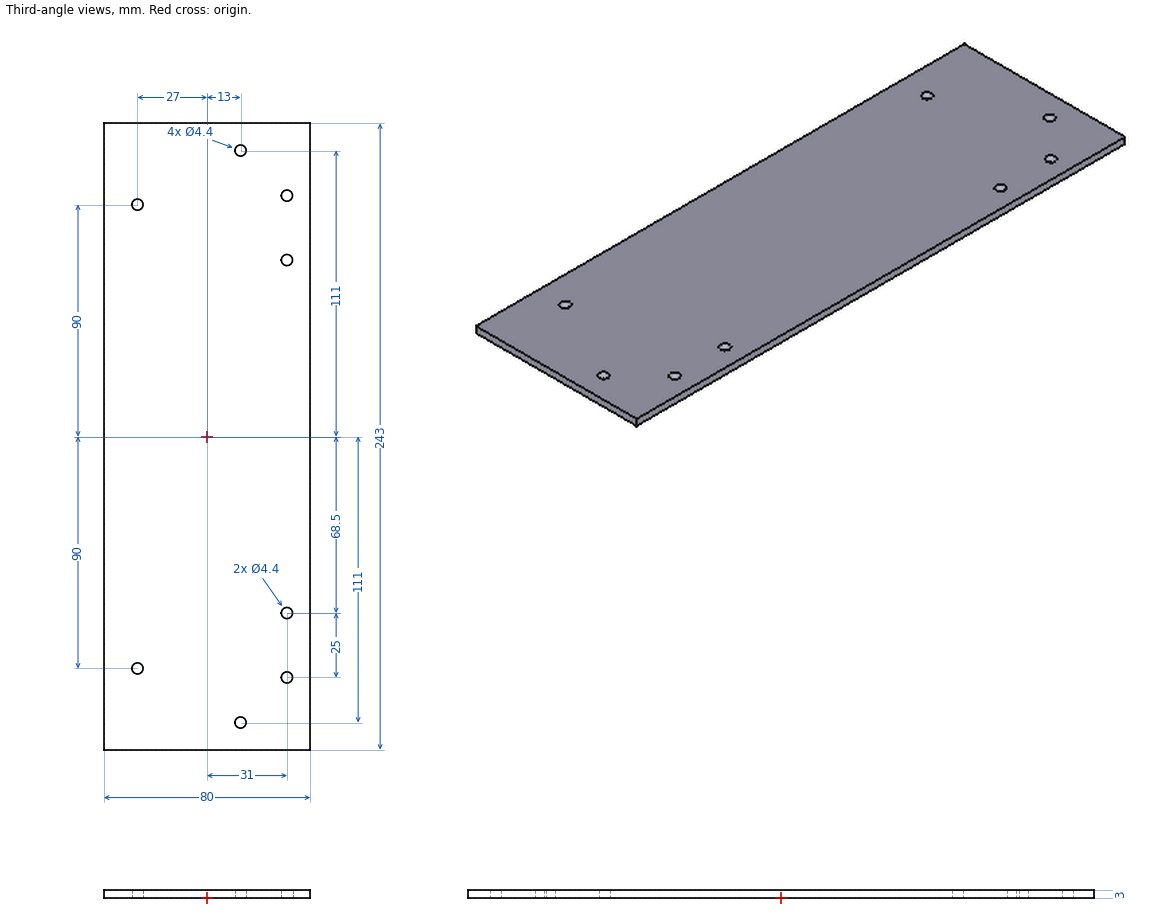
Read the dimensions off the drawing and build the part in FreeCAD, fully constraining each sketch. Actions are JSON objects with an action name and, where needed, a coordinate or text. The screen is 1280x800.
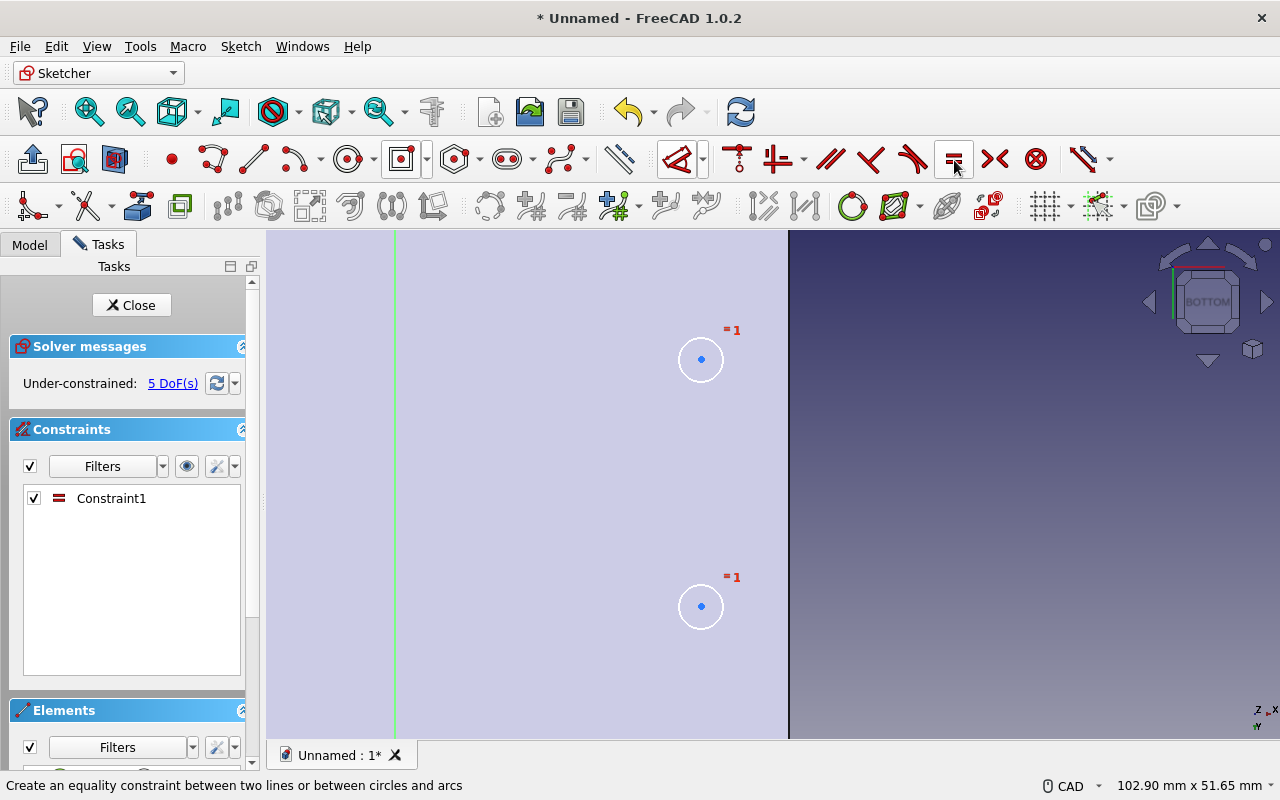
{"action": "left_click", "coordinate": [701, 607]}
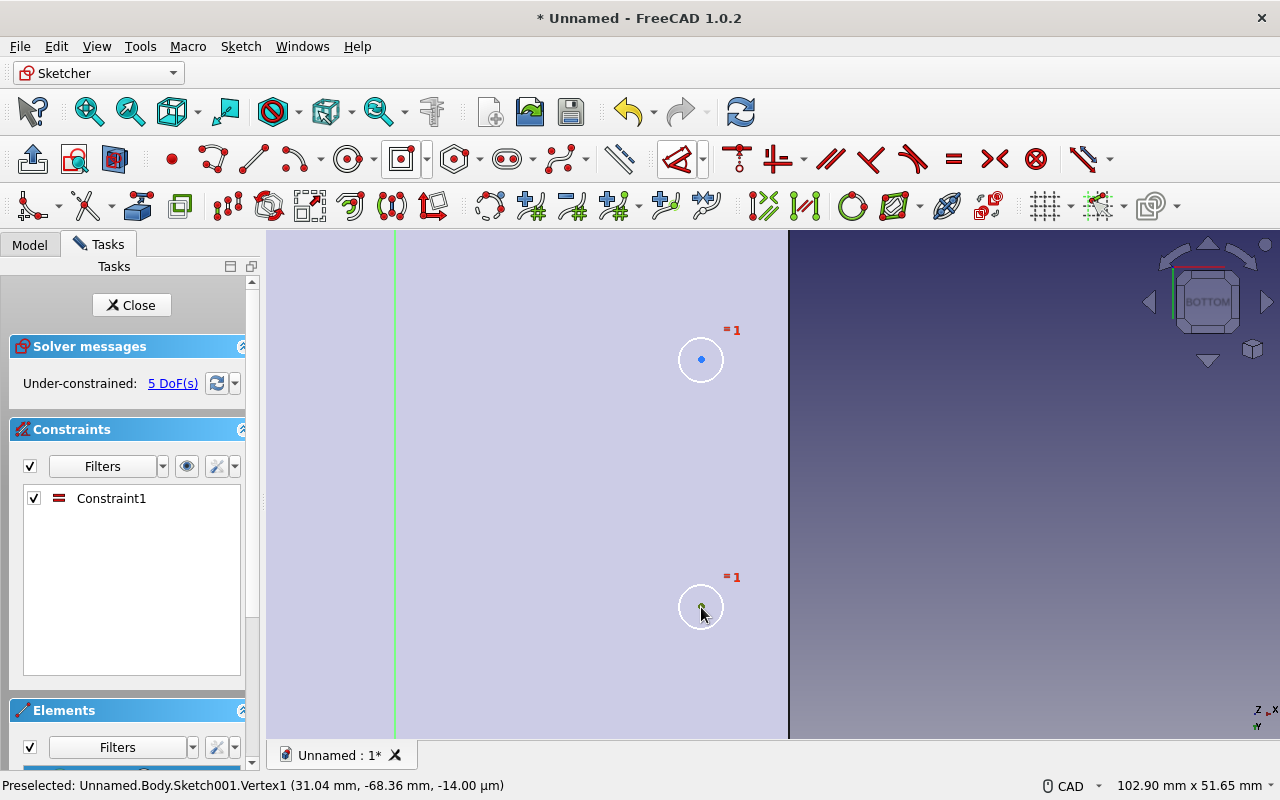
{"action": "left_click", "coordinate": [701, 360]}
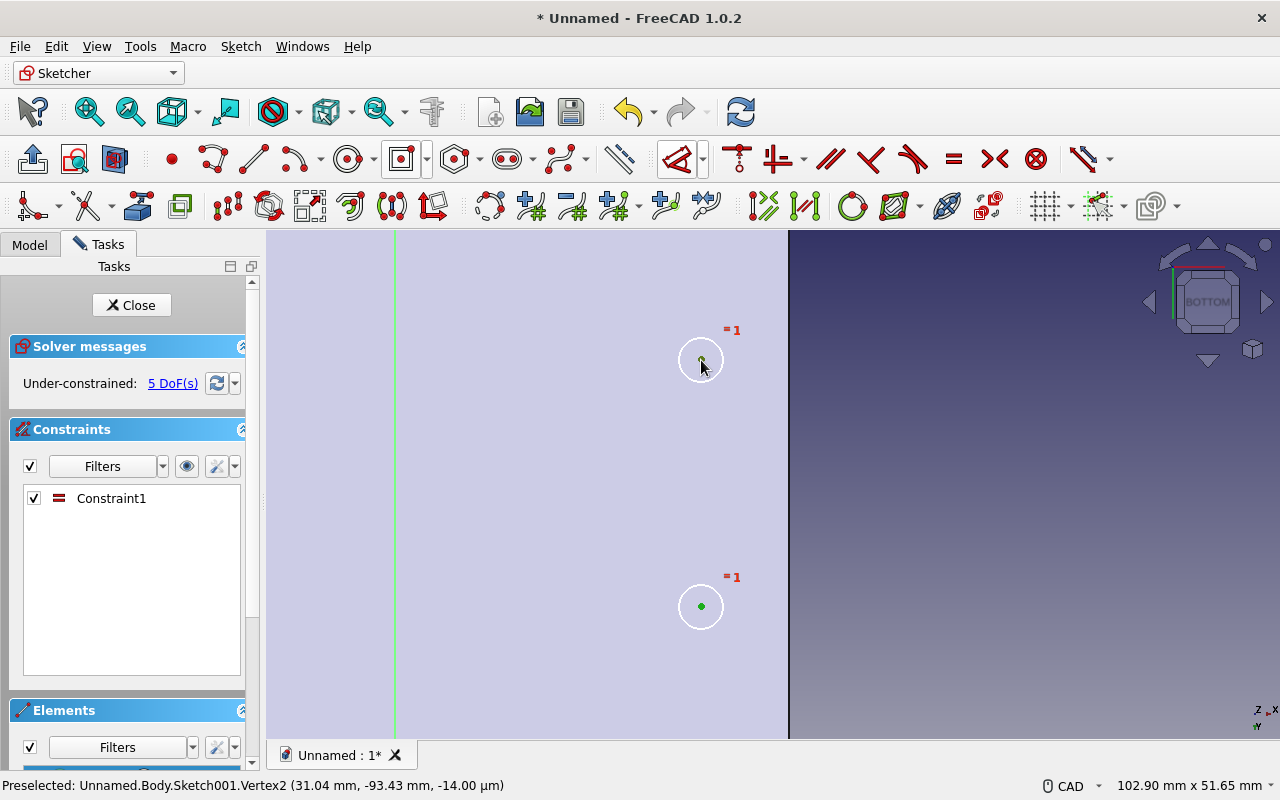
{"action": "left_click", "coordinate": [804, 160]}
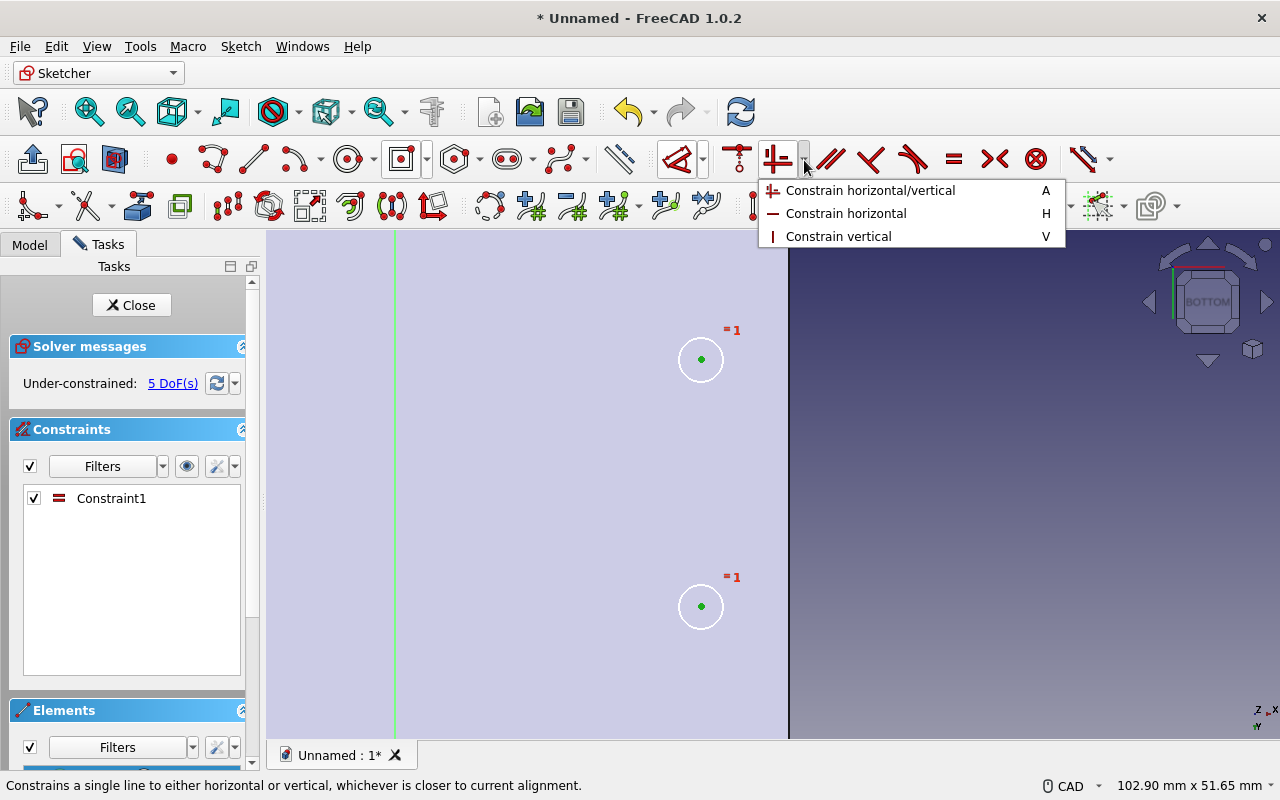
{"action": "left_click", "coordinate": [912, 236]}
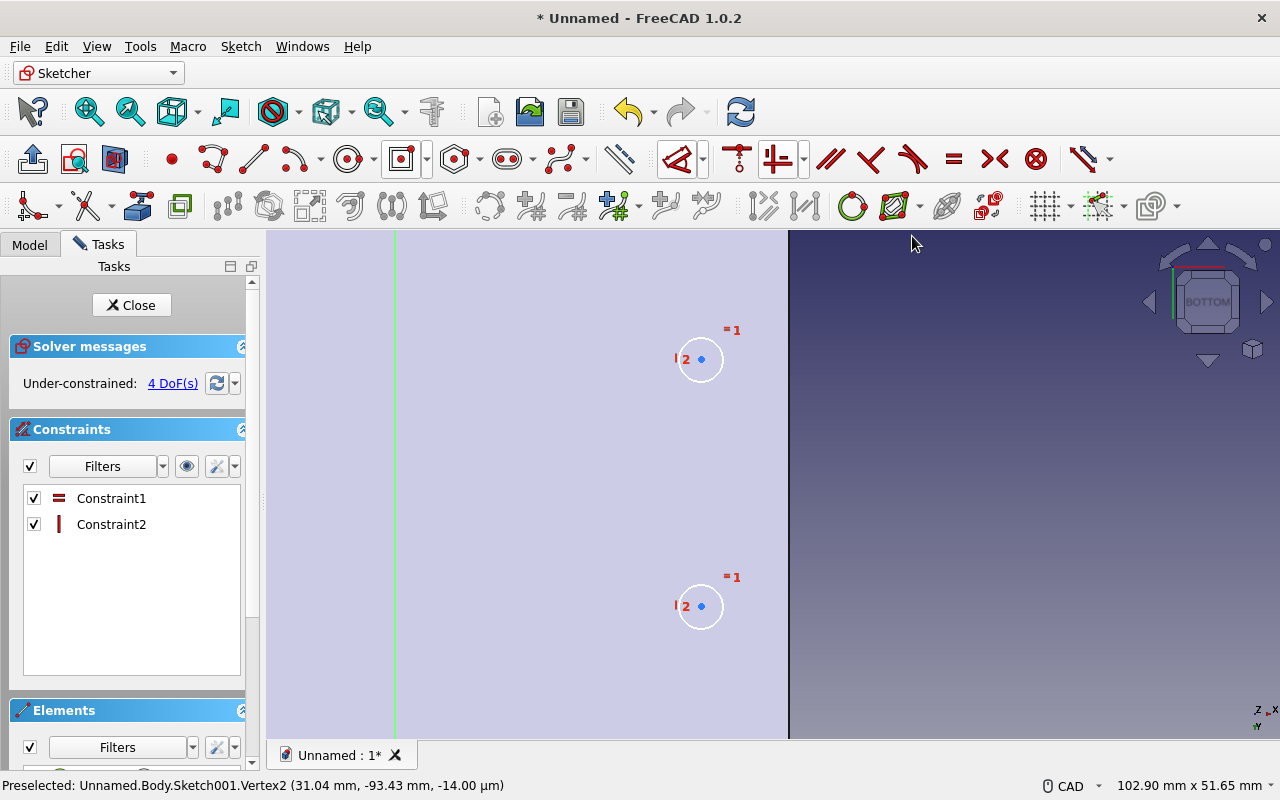
{"action": "left_click", "coordinate": [716, 591]}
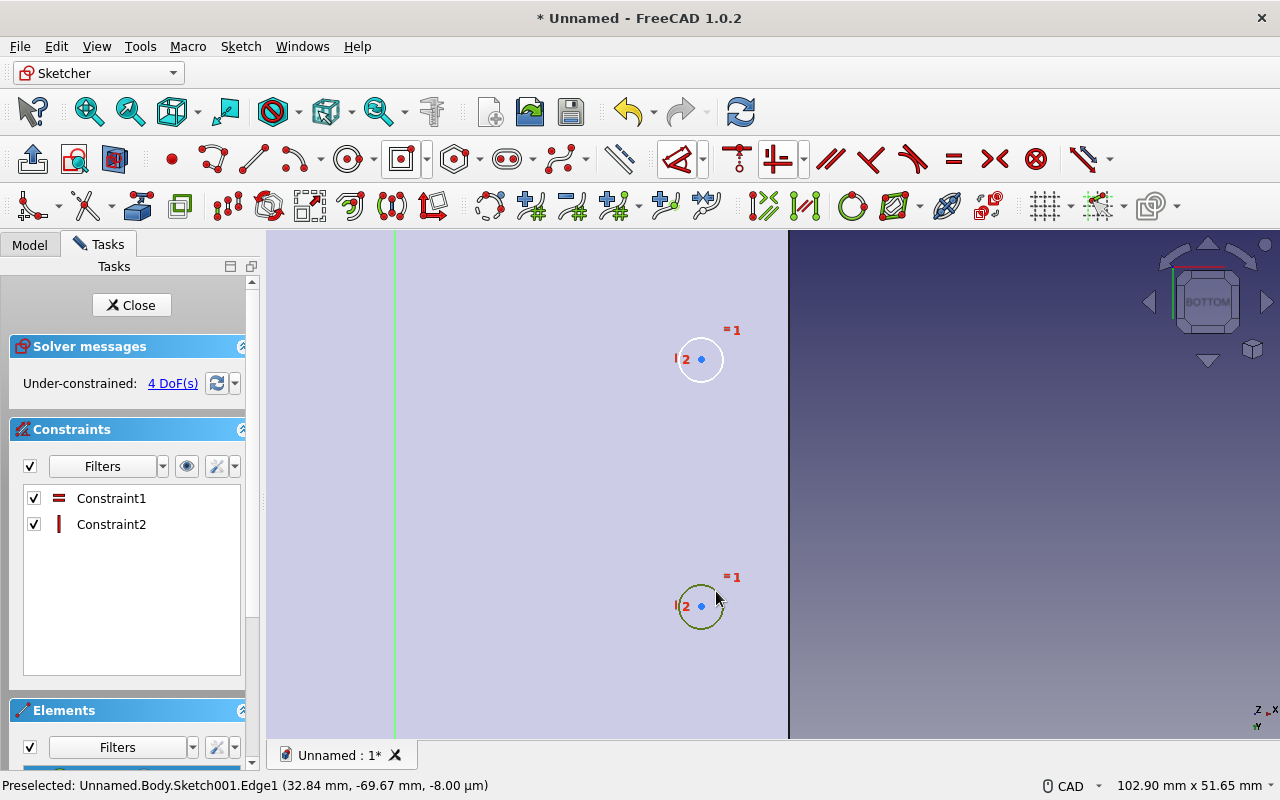
{"action": "left_click", "coordinate": [702, 160]}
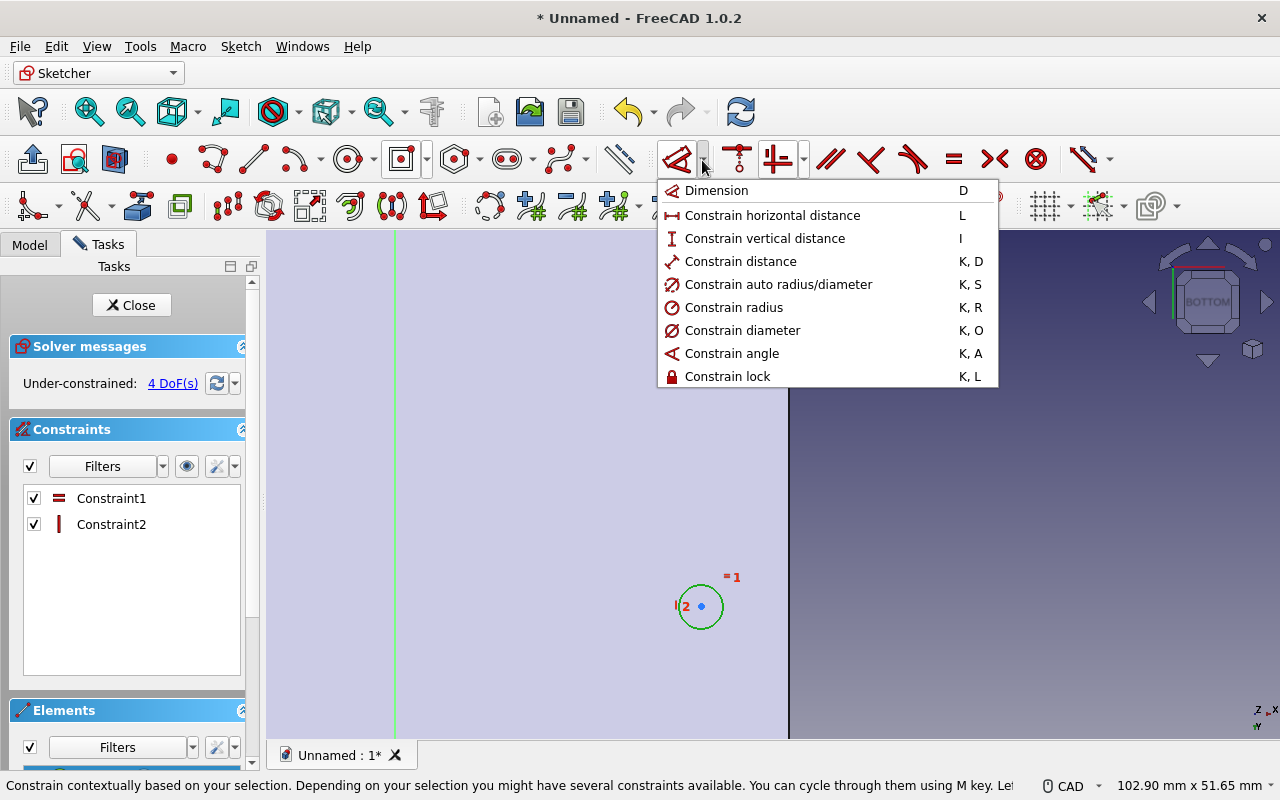
{"action": "left_click", "coordinate": [828, 330]}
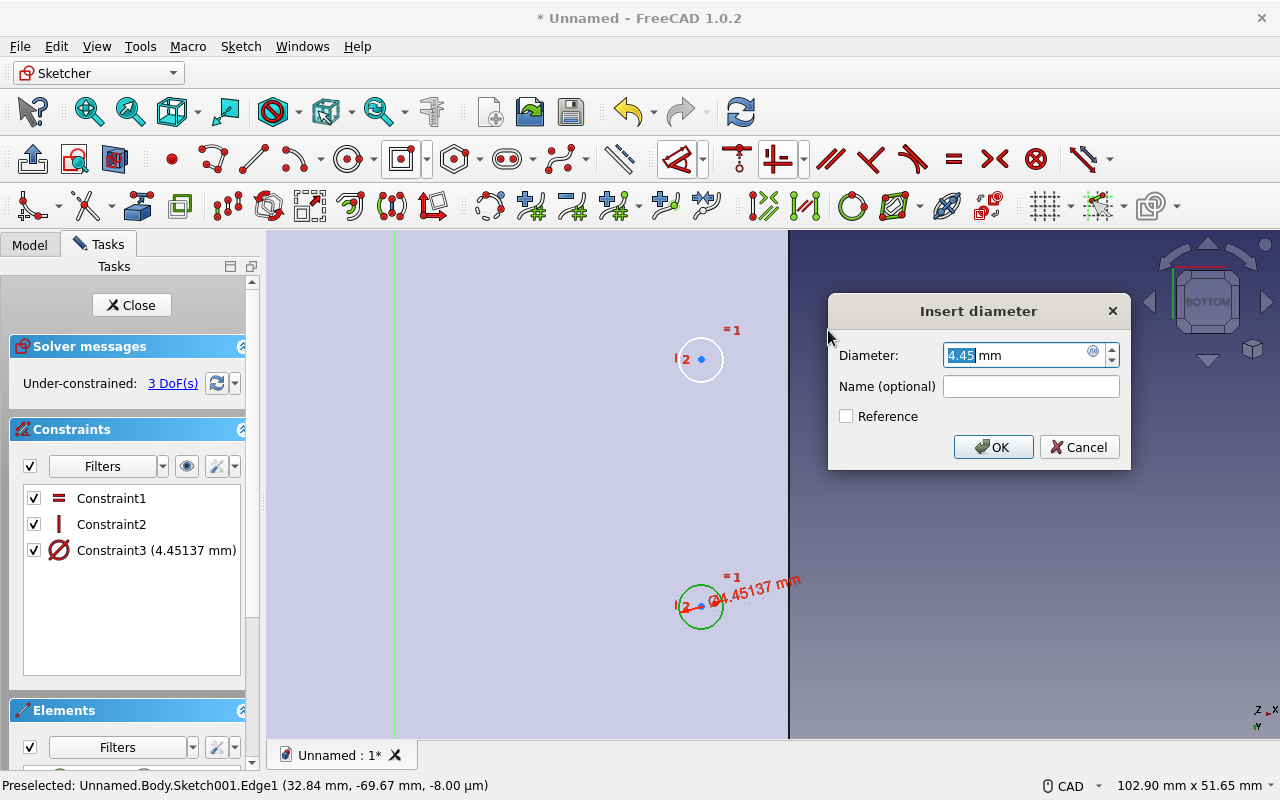
{"action": "type", "text": "4.4"}
{"action": "key", "text": "Return"}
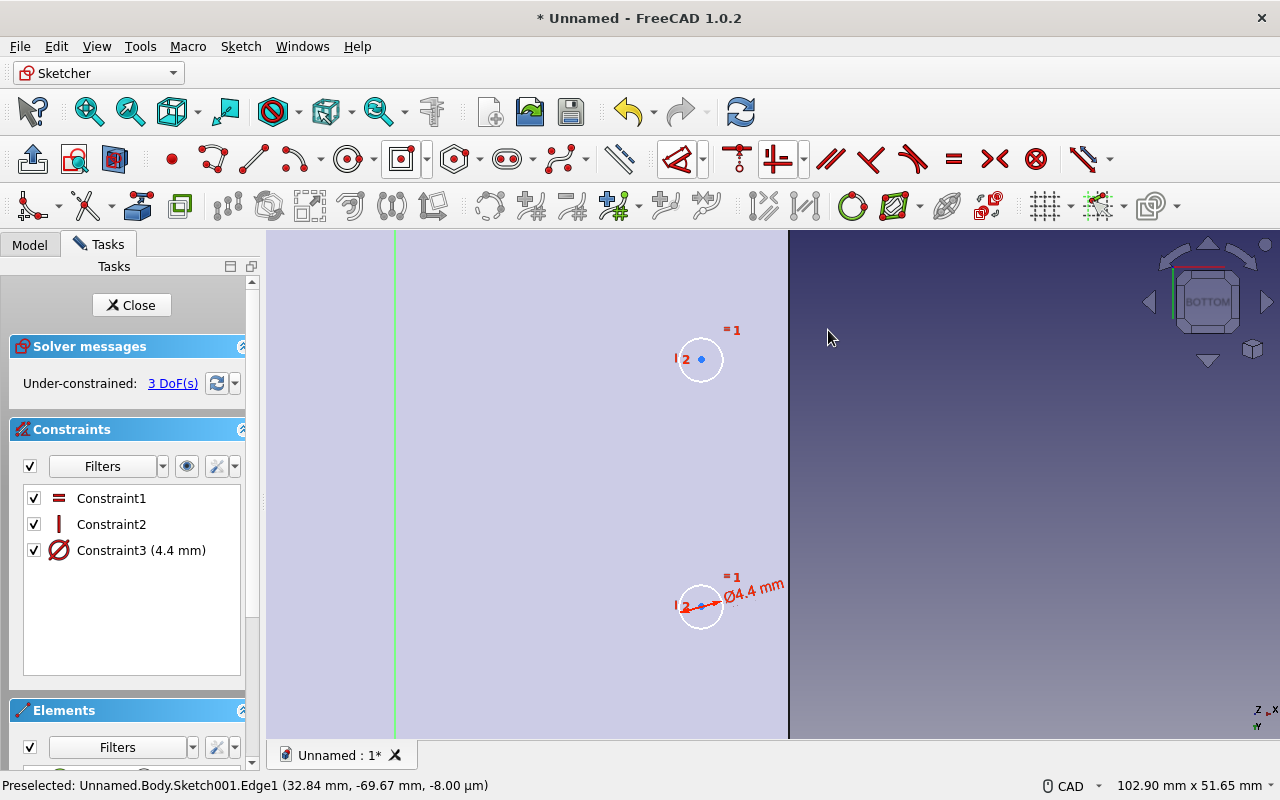
{"action": "left_click", "coordinate": [701, 607]}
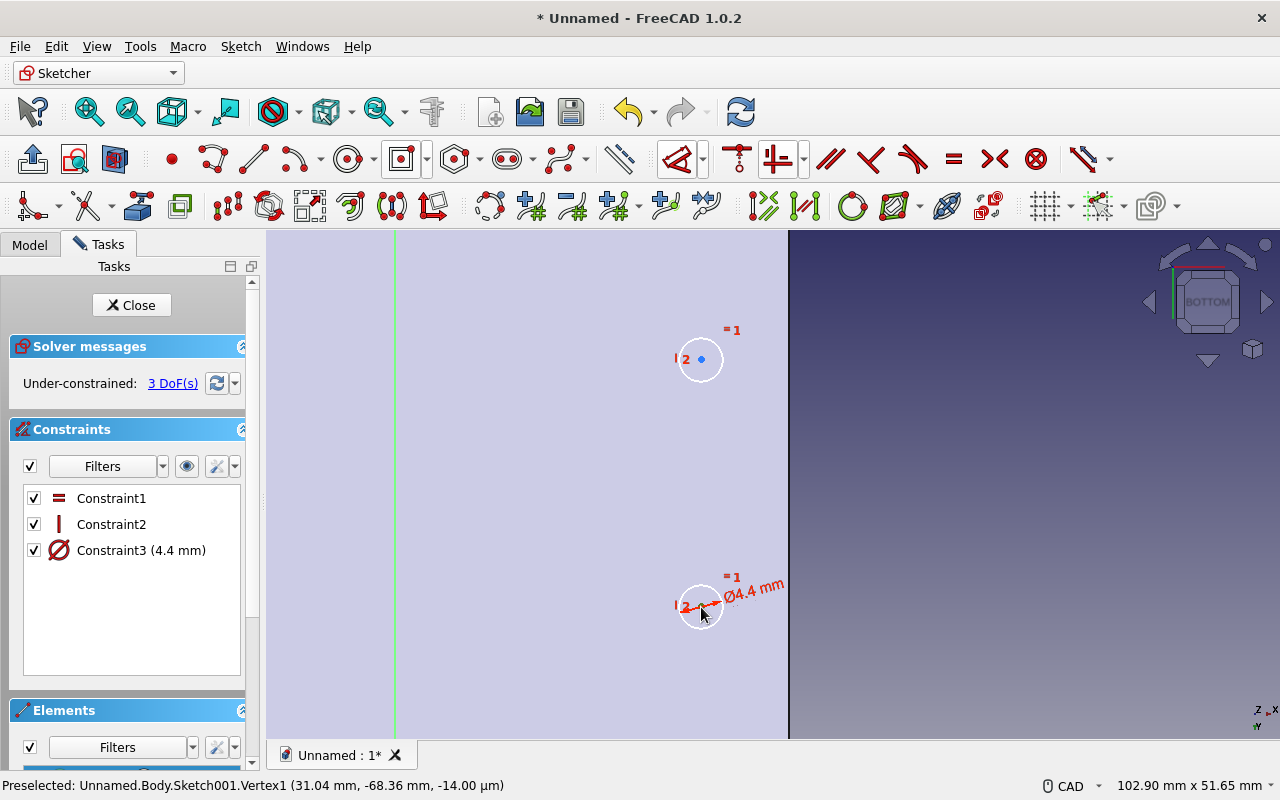
{"action": "key", "text": "l"}